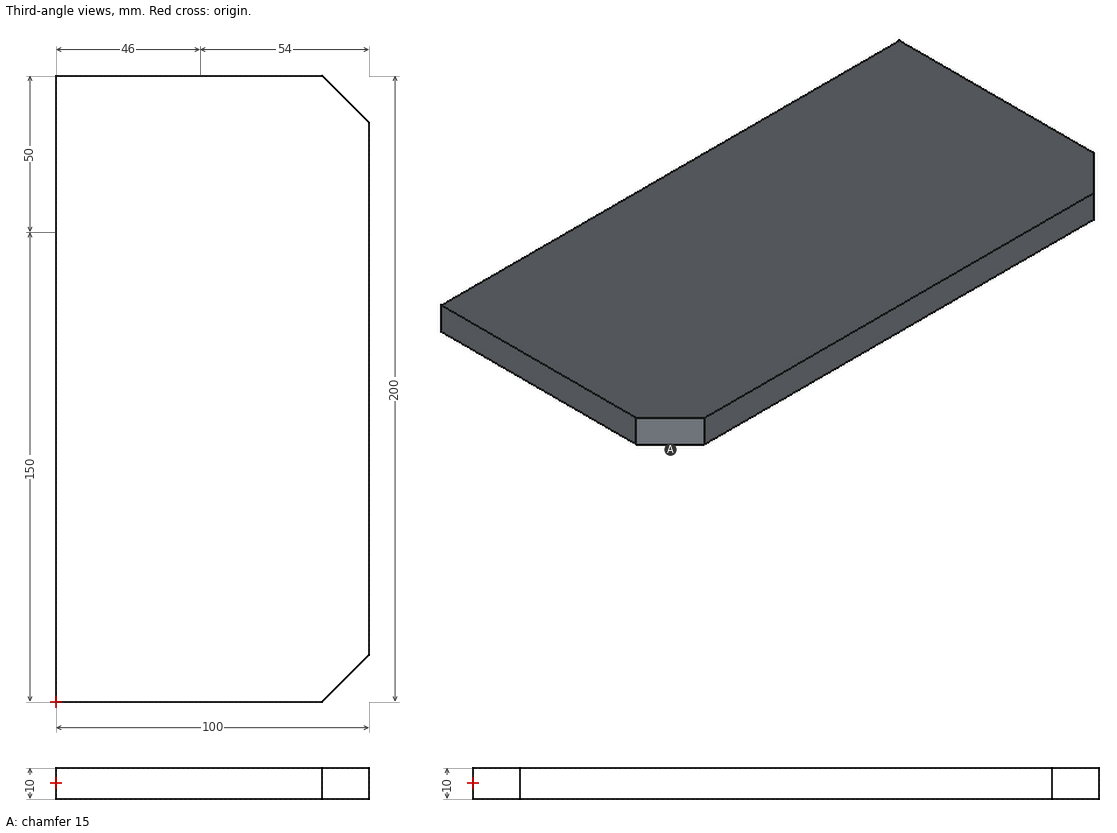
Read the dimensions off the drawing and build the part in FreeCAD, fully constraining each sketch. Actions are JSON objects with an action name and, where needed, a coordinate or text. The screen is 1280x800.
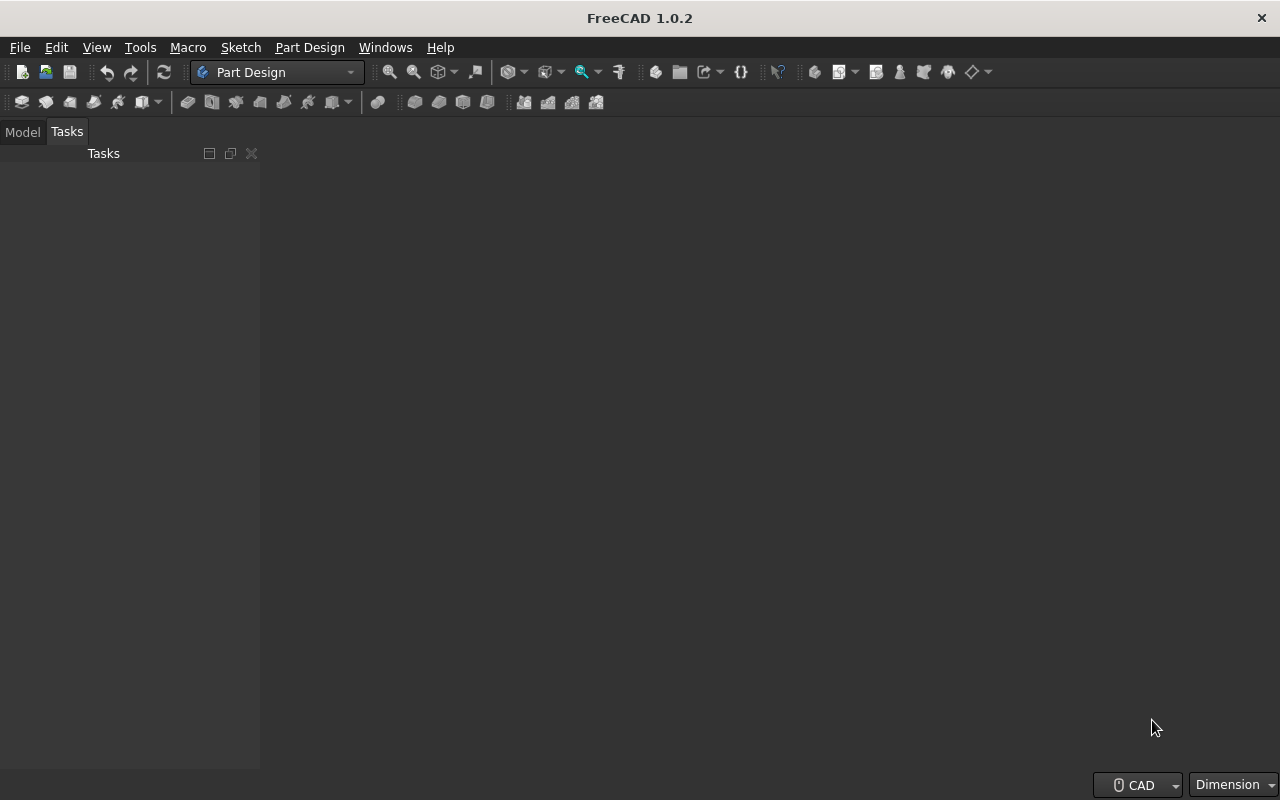
{"action": "key", "text": "ctrl+n"}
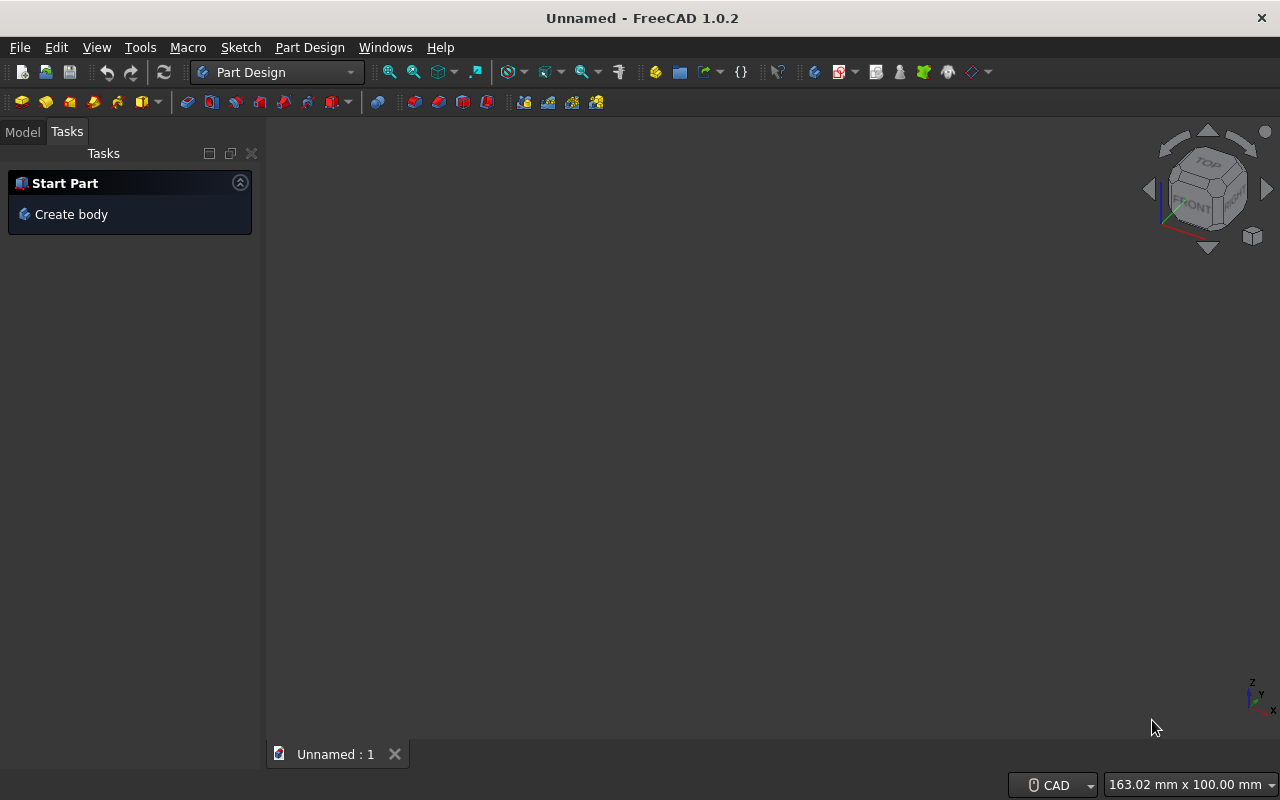
{"action": "left_click", "coordinate": [840, 72]}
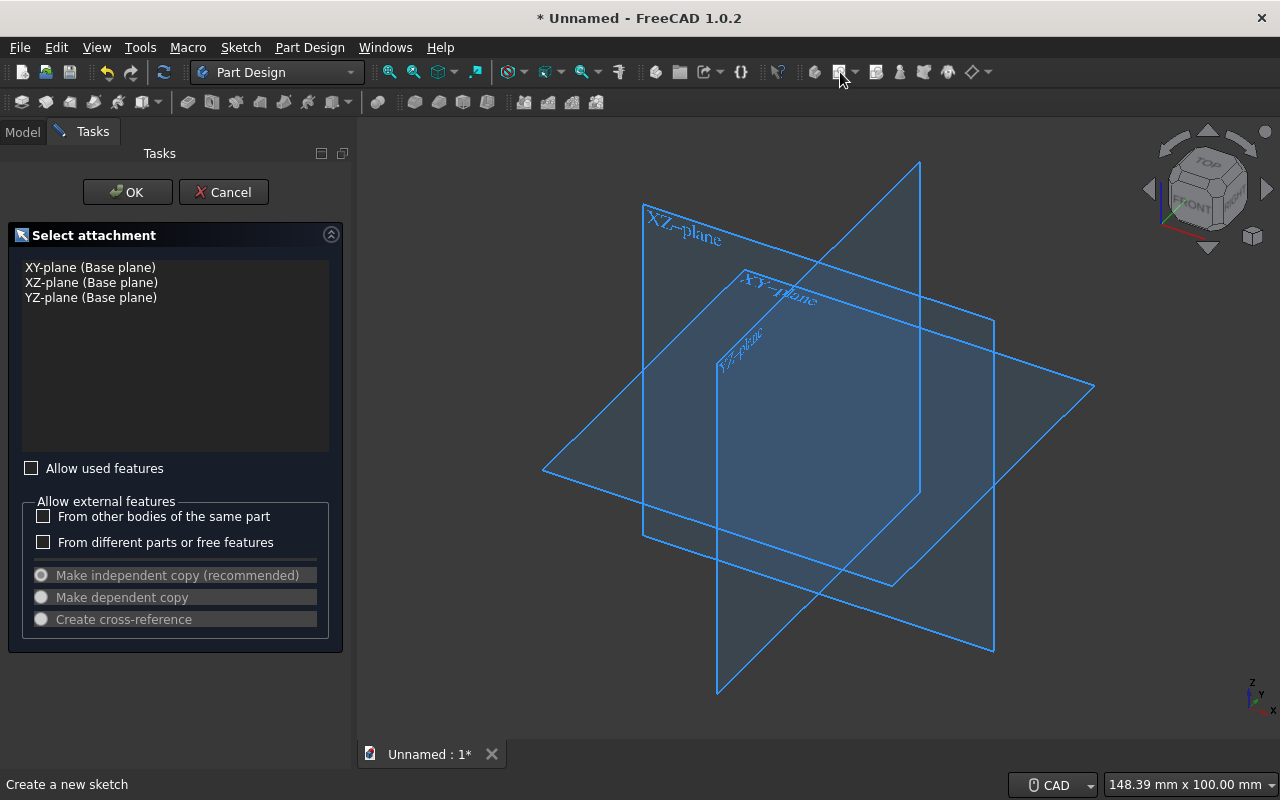
{"action": "left_click", "coordinate": [82, 268]}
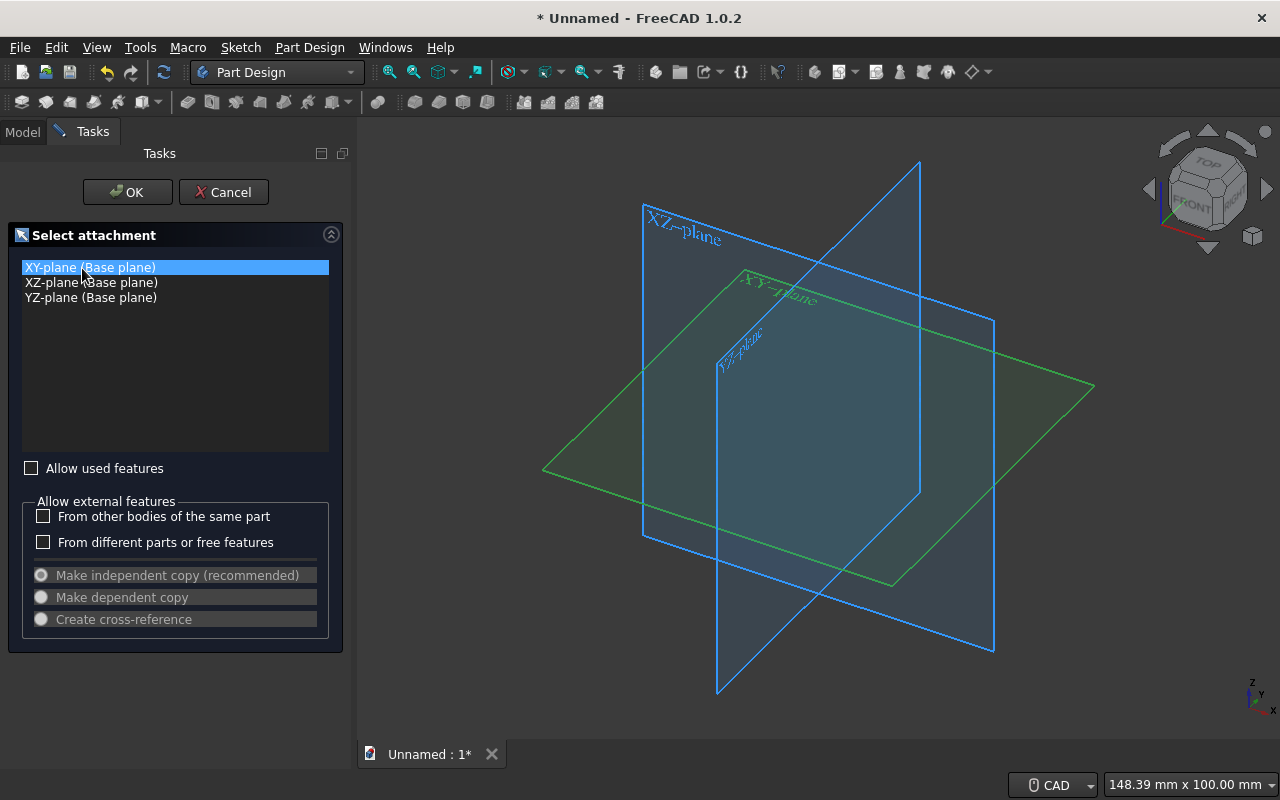
{"action": "left_click", "coordinate": [128, 192]}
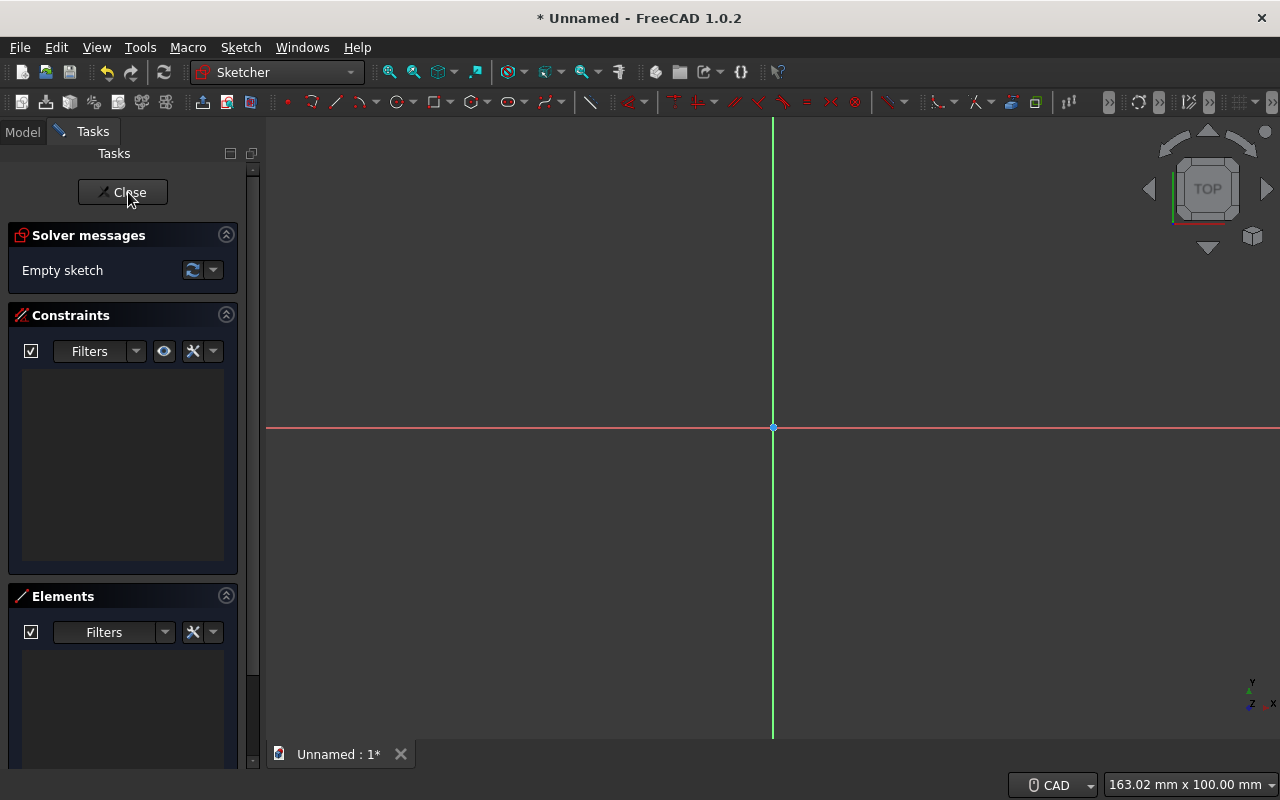
{"action": "scroll", "coordinate": [541, 696], "scroll_direction": "down", "scroll_amount": 6}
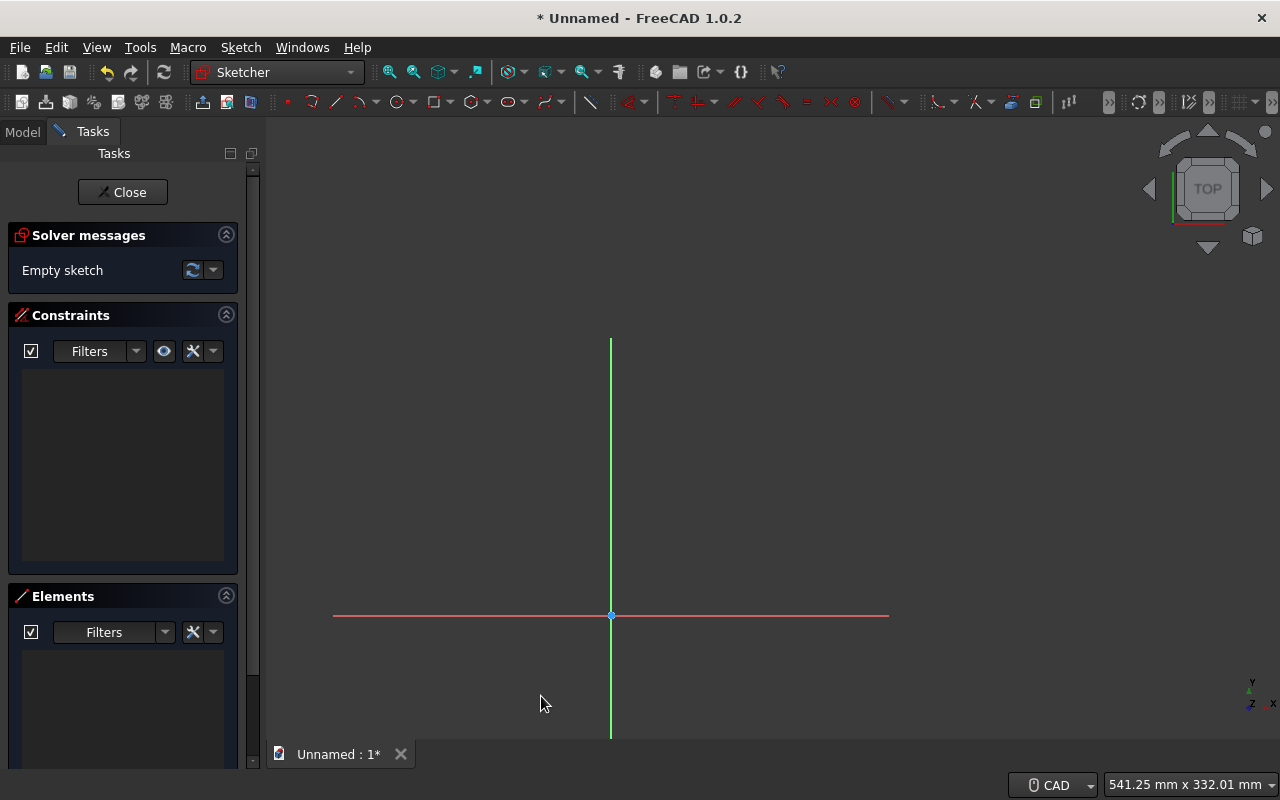
{"action": "left_click", "coordinate": [312, 102]}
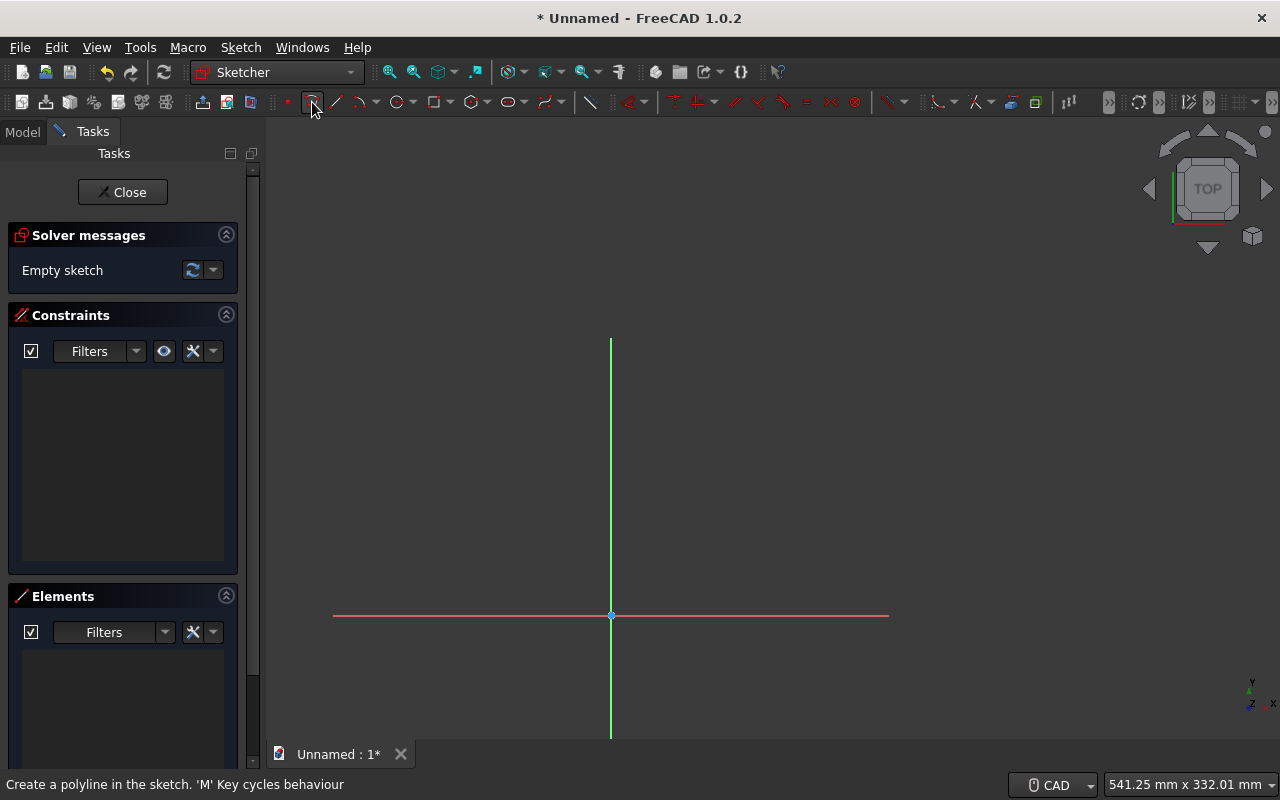
{"action": "left_click", "coordinate": [611, 616]}
{"action": "left_click", "coordinate": [798, 607]}
{"action": "left_click", "coordinate": [798, 241]}
{"action": "left_click", "coordinate": [697, 241]}
{"action": "left_click", "coordinate": [620, 335]}
{"action": "left_click", "coordinate": [611, 616]}
{"action": "key", "text": "Escape"}
{"action": "key", "text": "Escape"}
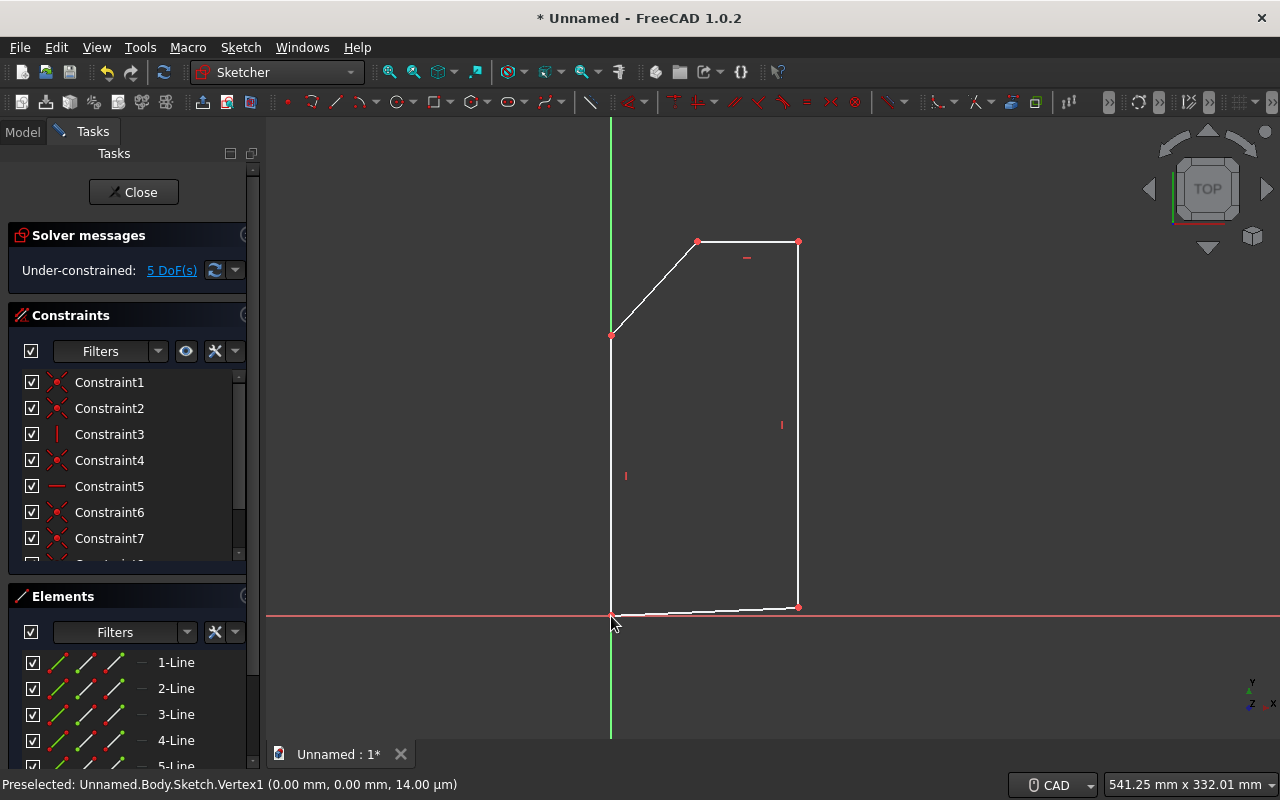
{"action": "left_click", "coordinate": [667, 614]}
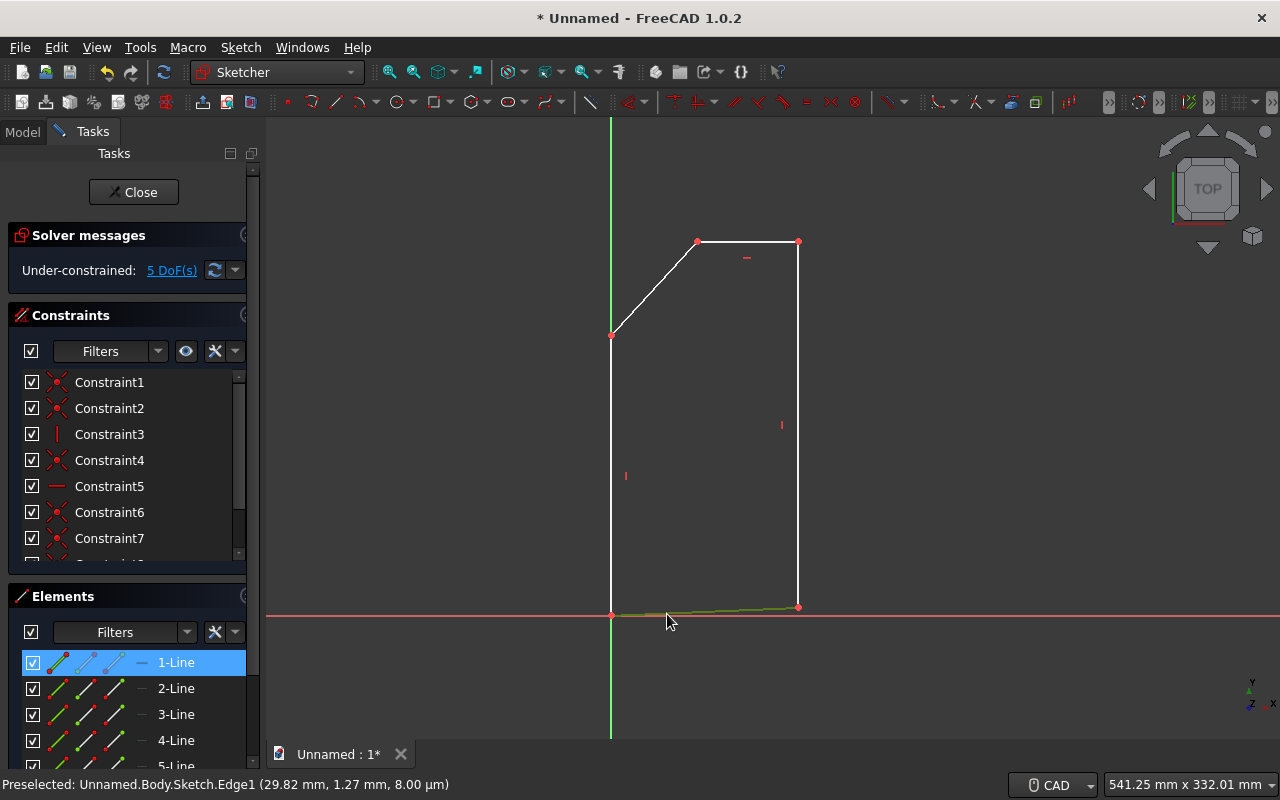
{"action": "key", "text": "h"}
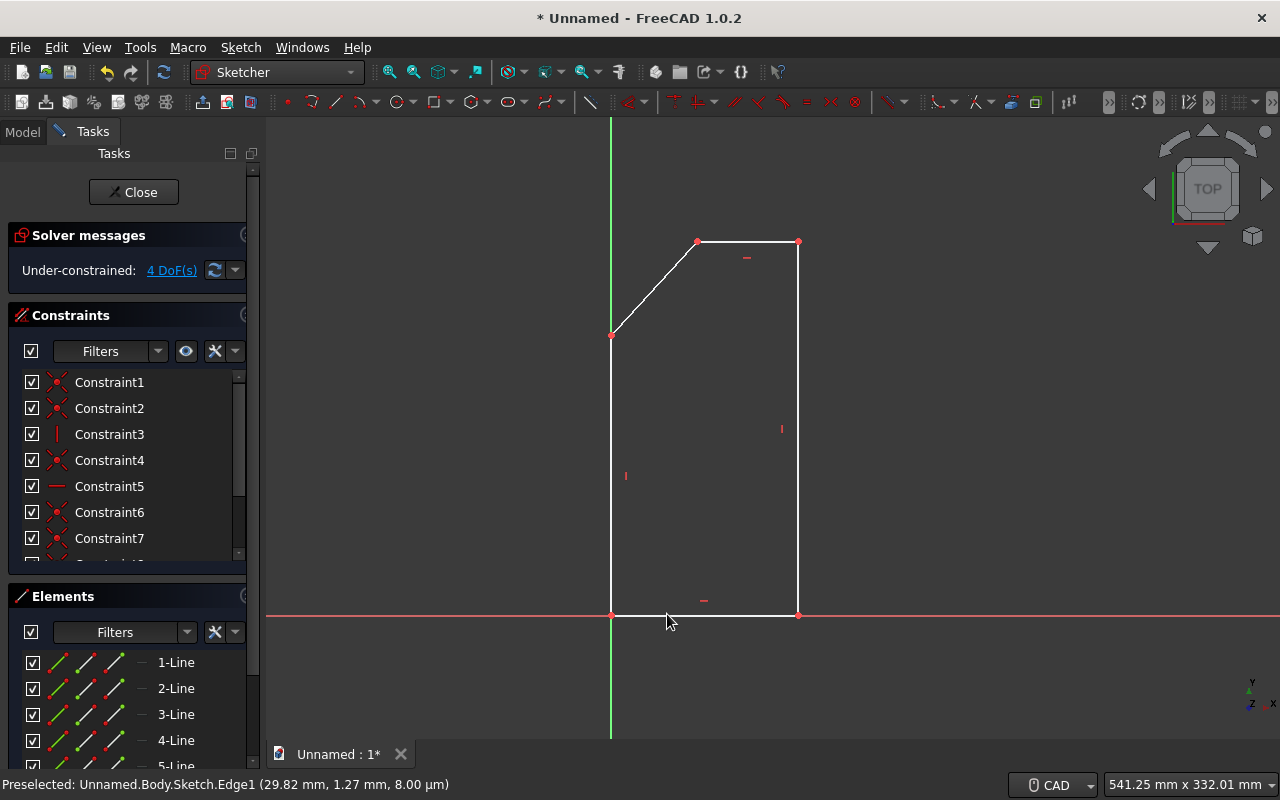
{"action": "key", "text": "d"}